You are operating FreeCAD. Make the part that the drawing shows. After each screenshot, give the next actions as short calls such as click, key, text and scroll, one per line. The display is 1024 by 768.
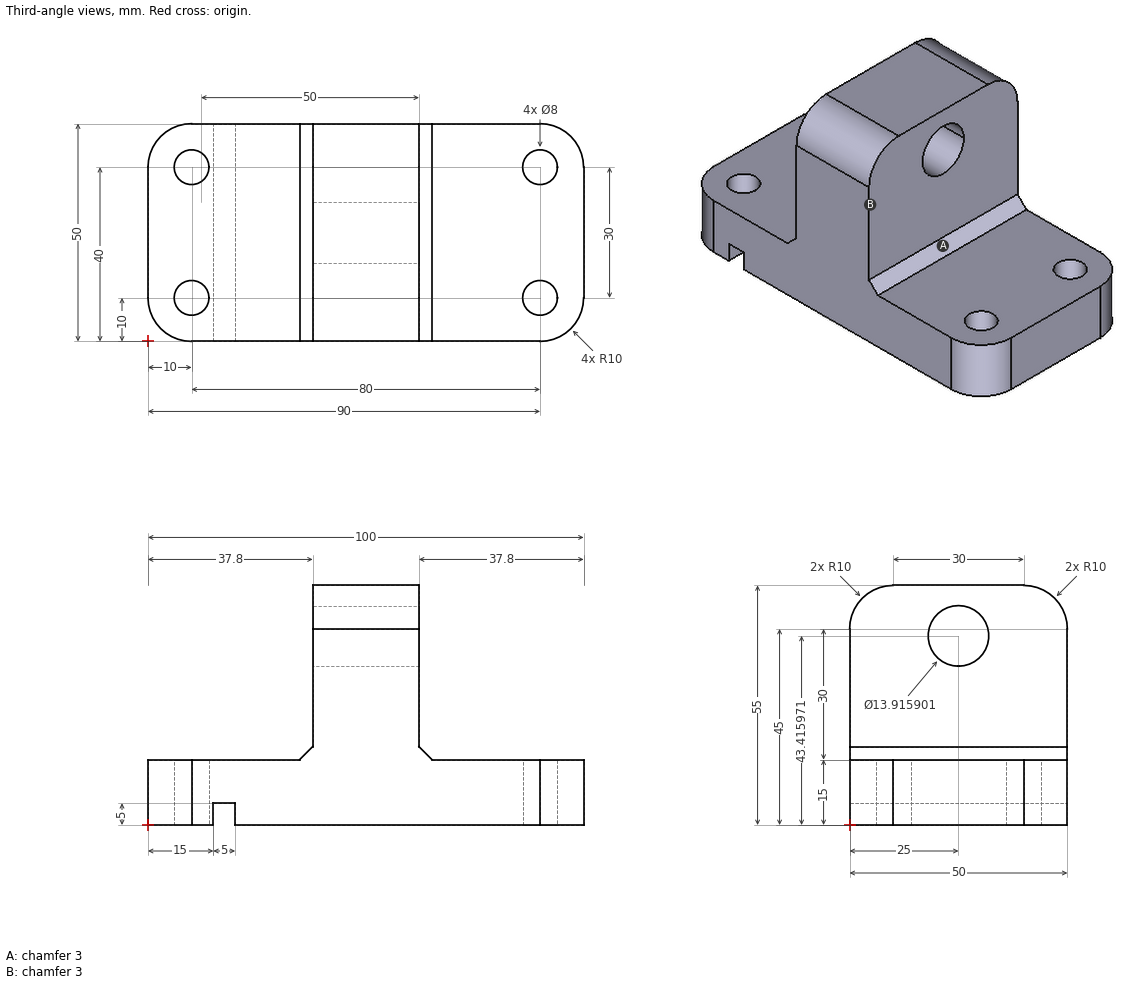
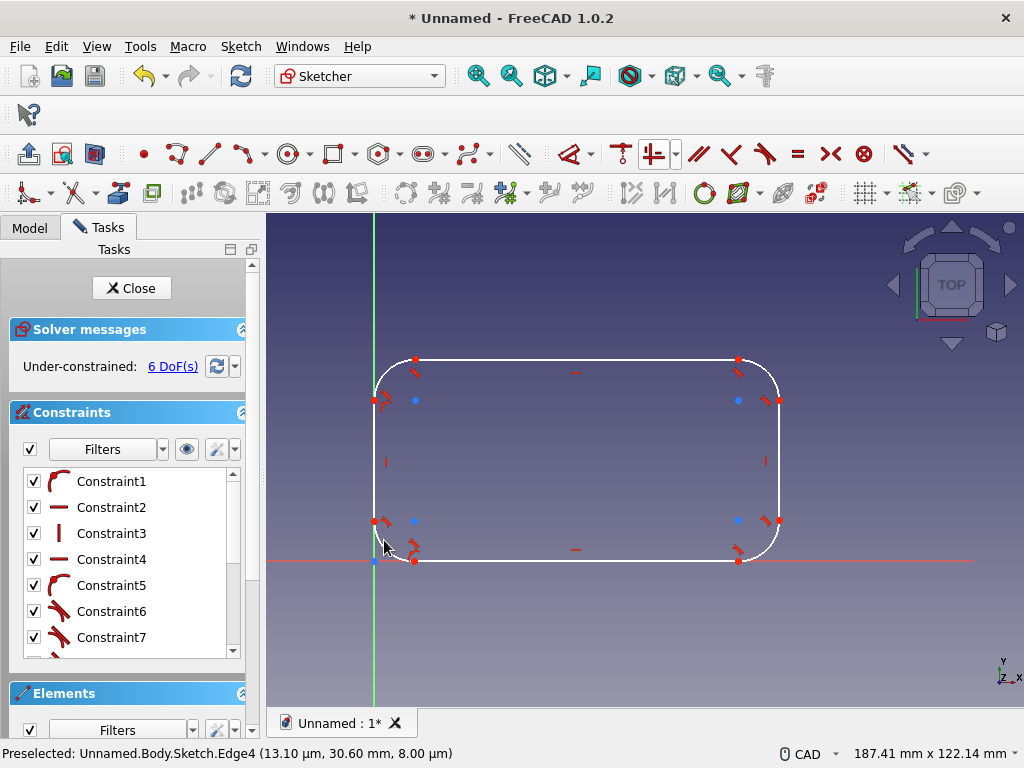
click(775, 539)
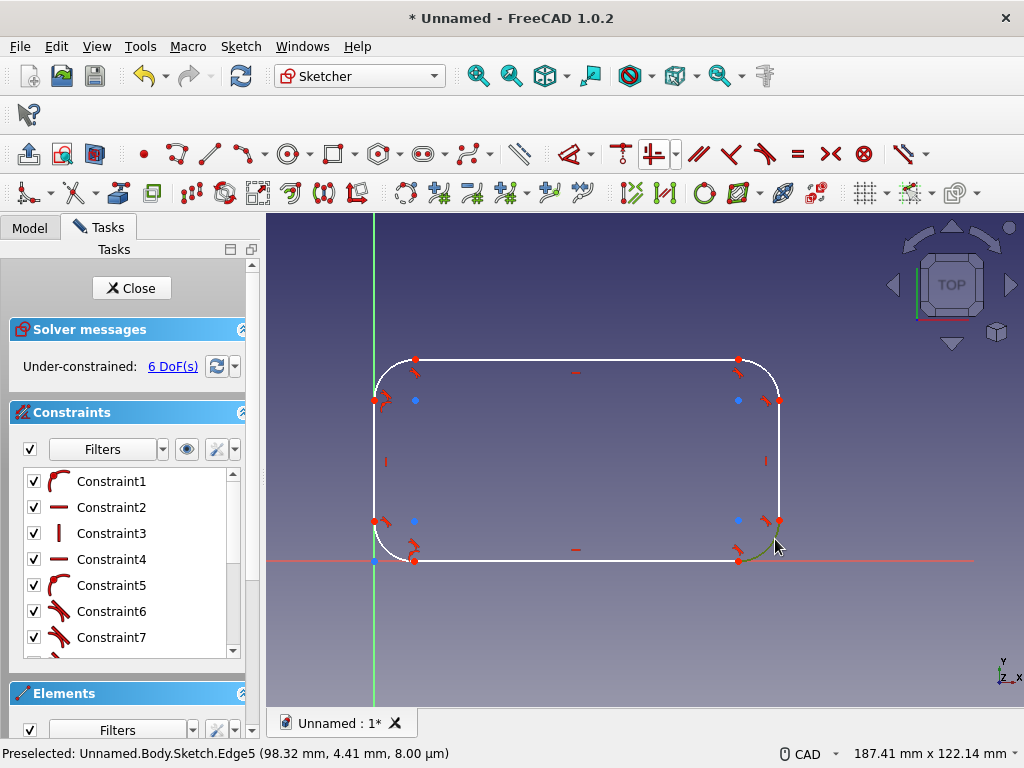
click(775, 382)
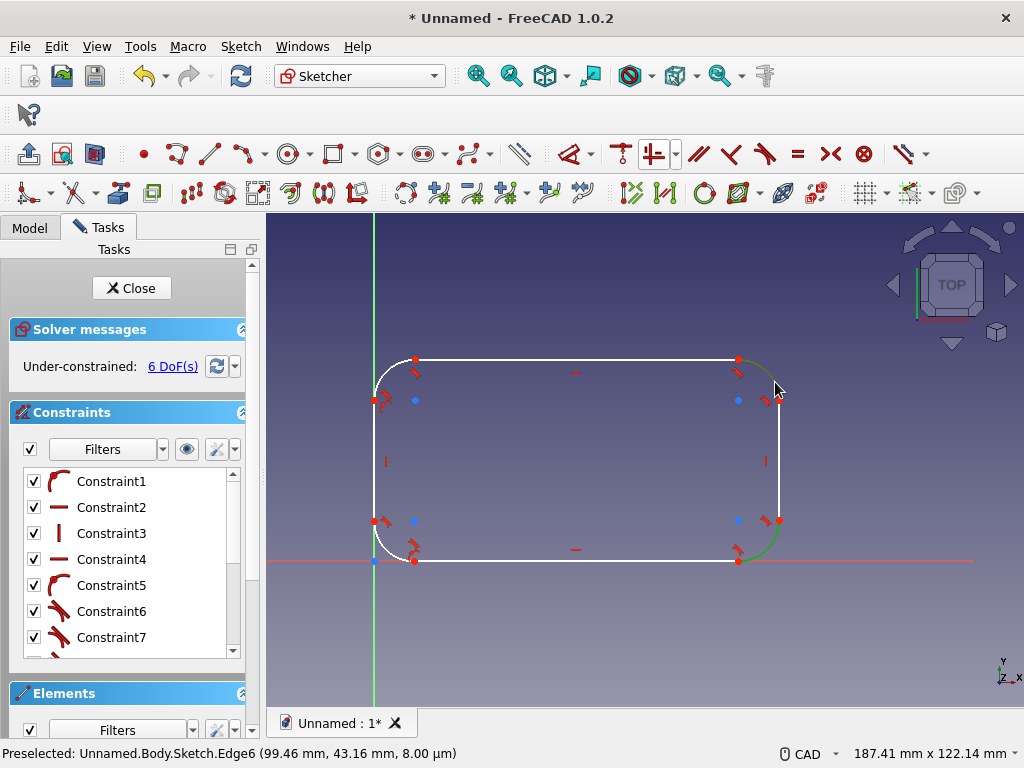
click(397, 364)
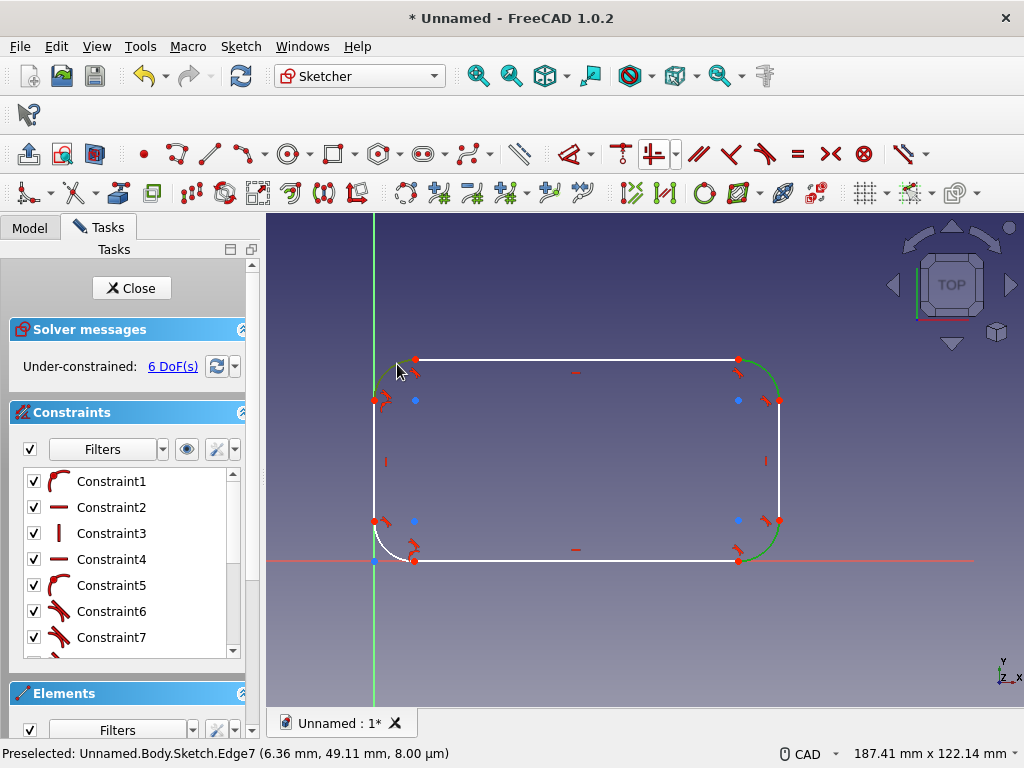
click(386, 550)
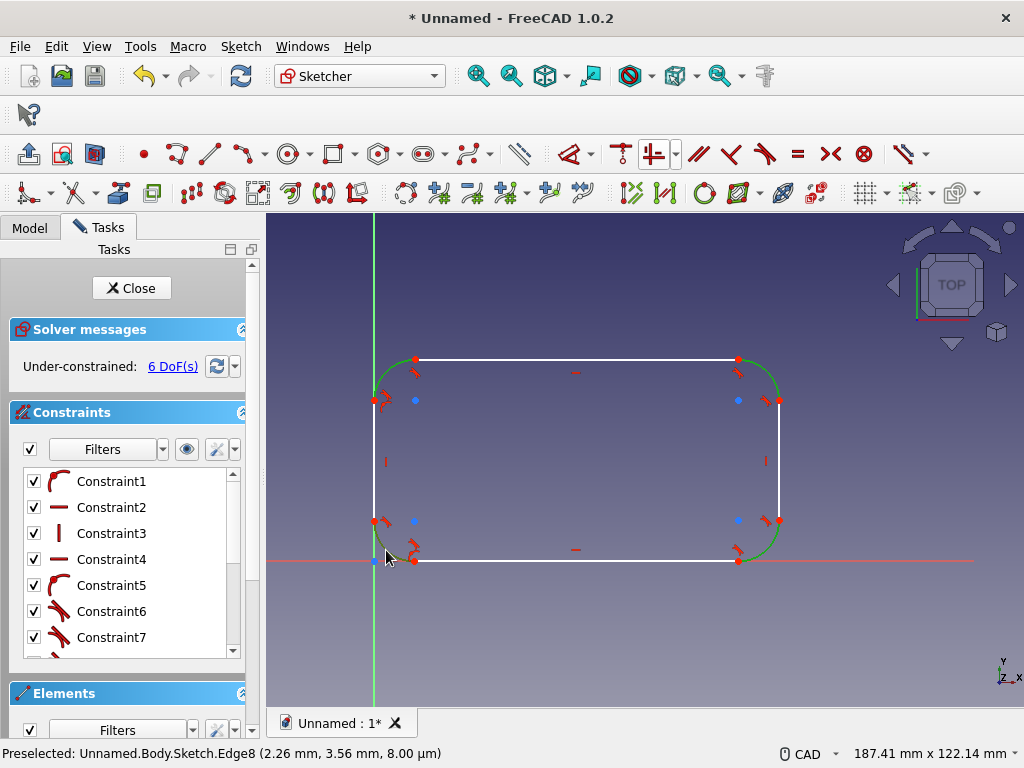
click(798, 154)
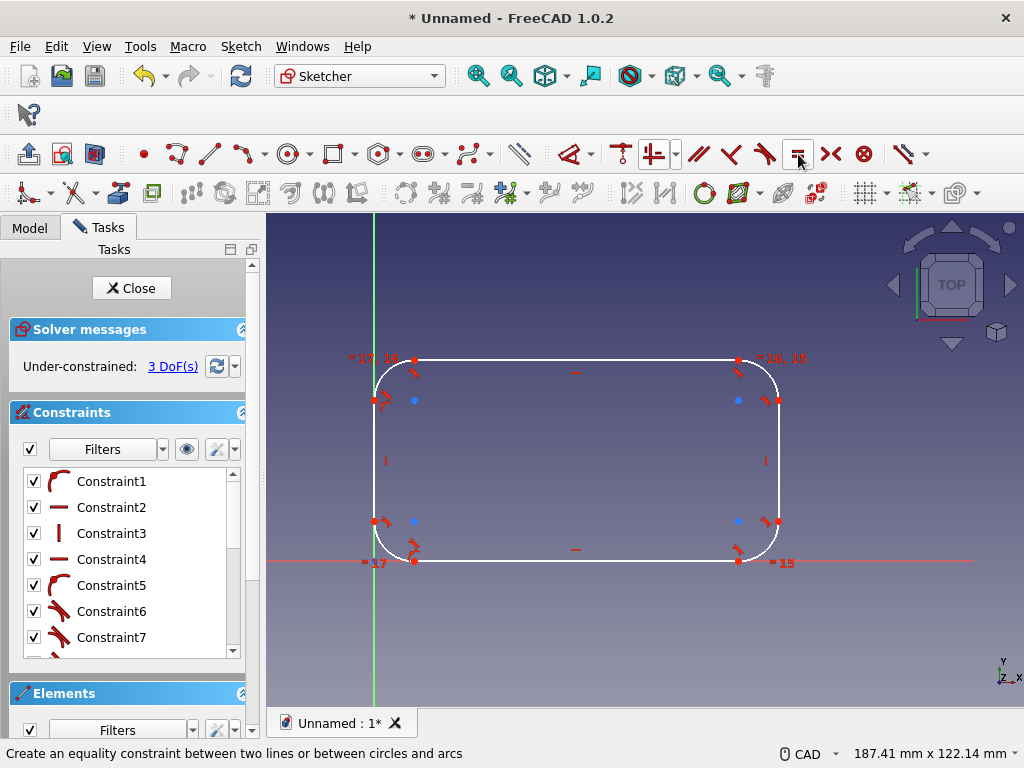
click(568, 154)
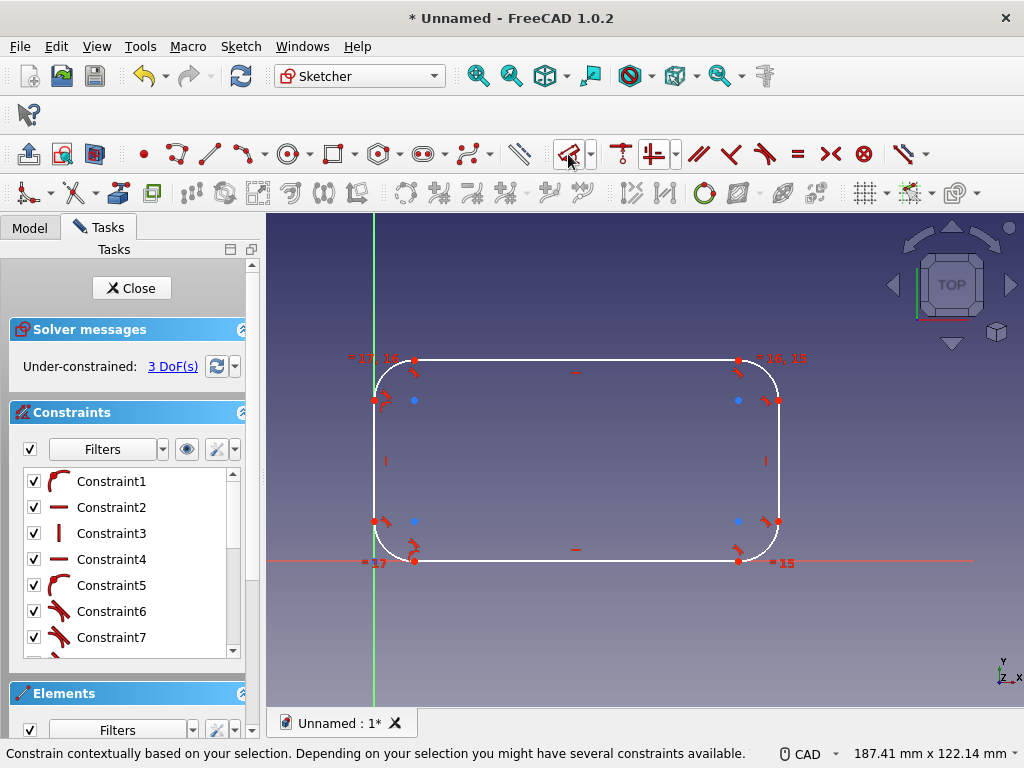
click(774, 539)
click(779, 580)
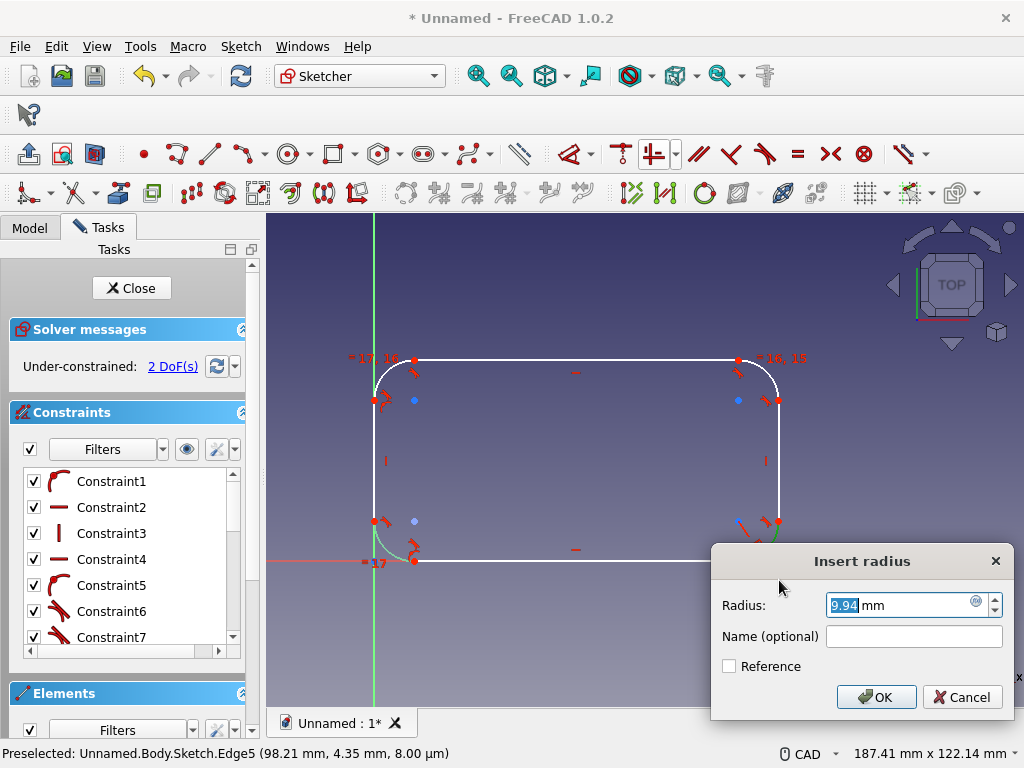
text(10)
key(Return)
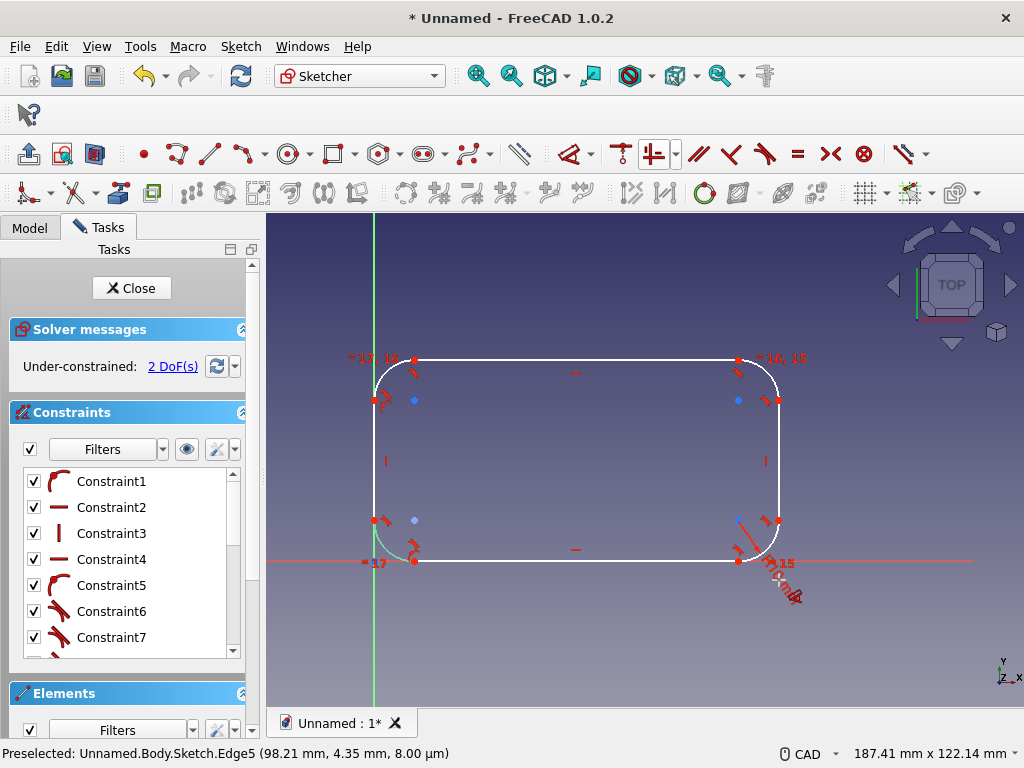
click(512, 561)
click(577, 595)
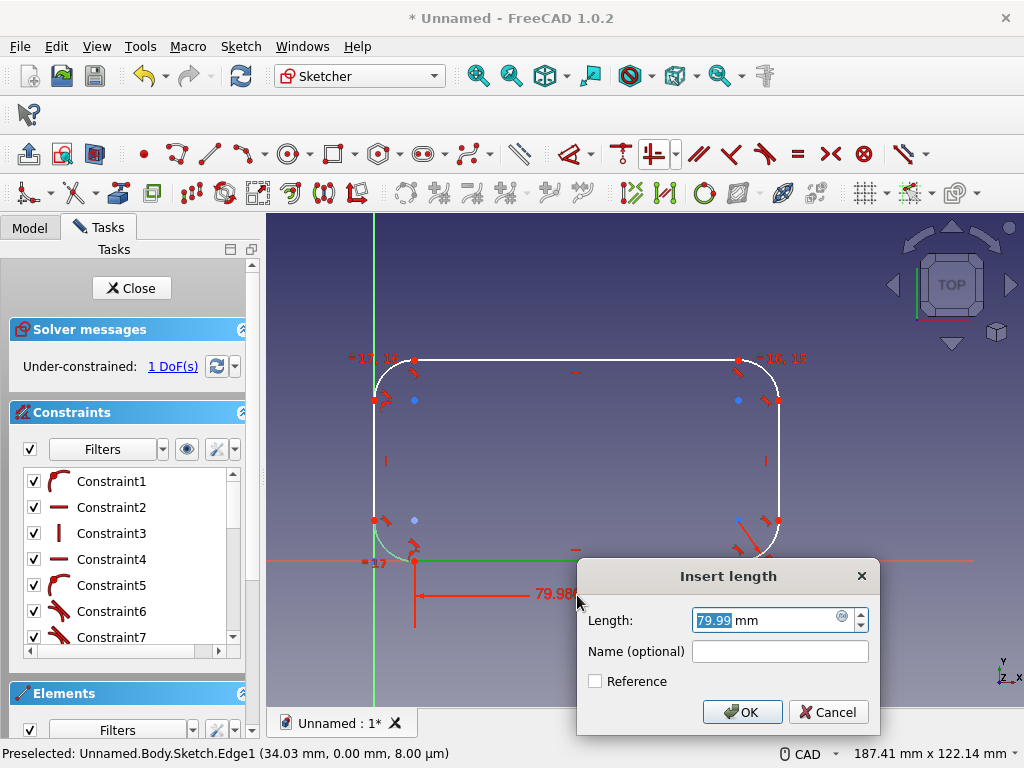
text(80)
key(Return)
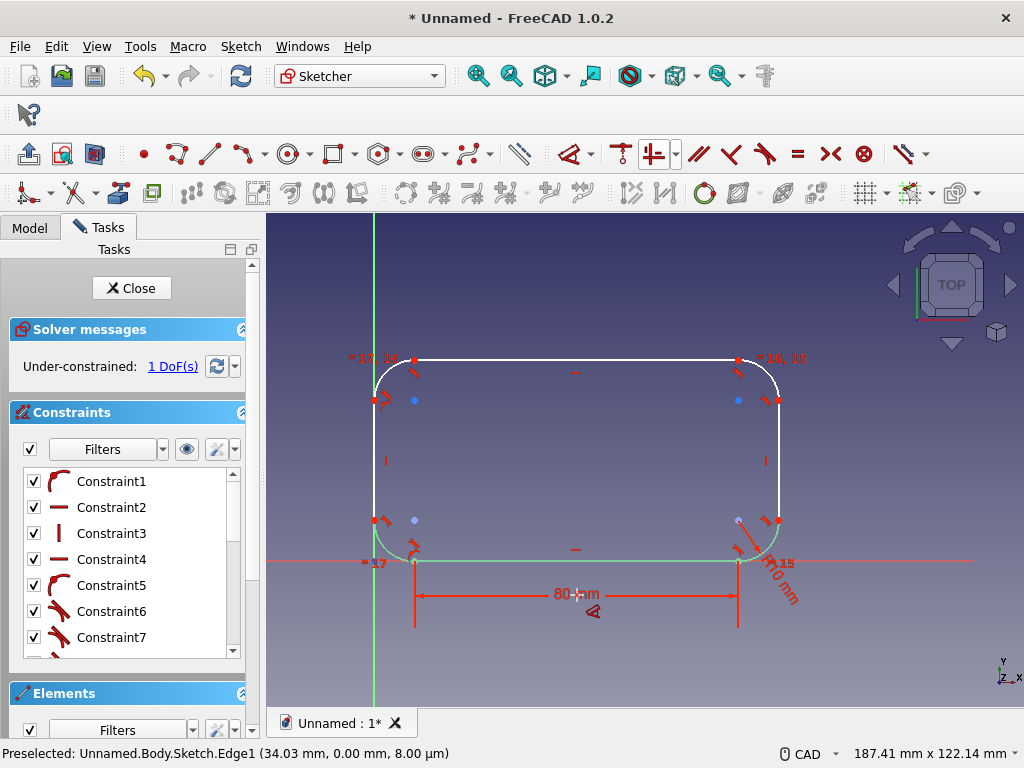
click(779, 485)
click(813, 461)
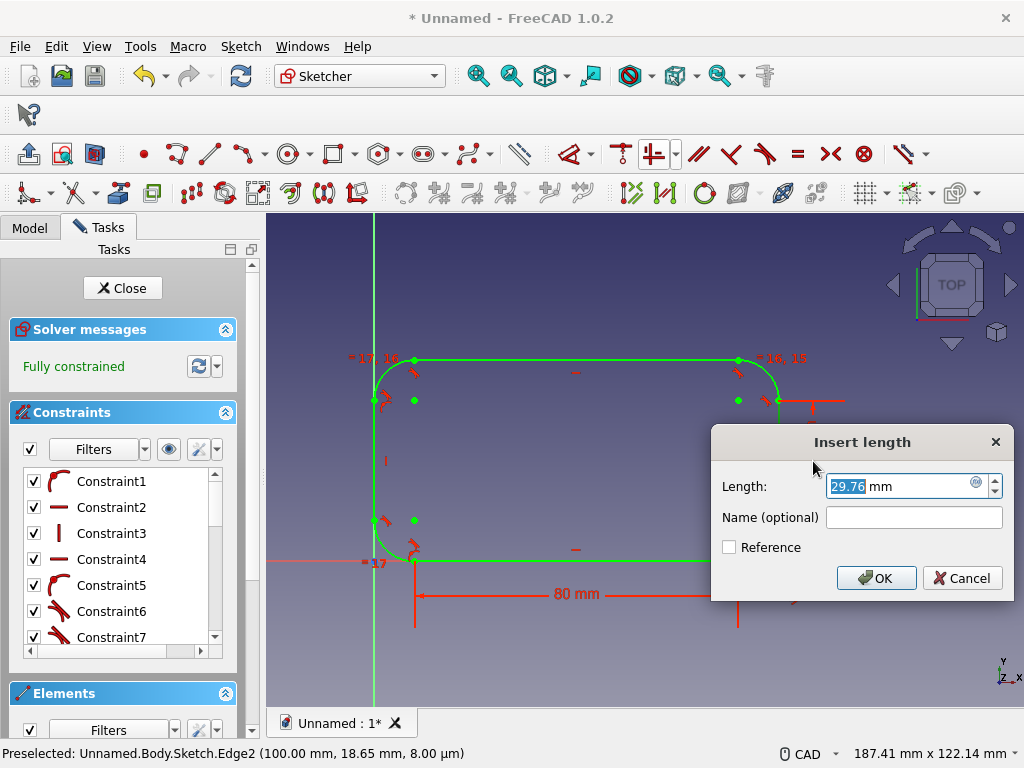
text(30)
key(Return)
key(Escape)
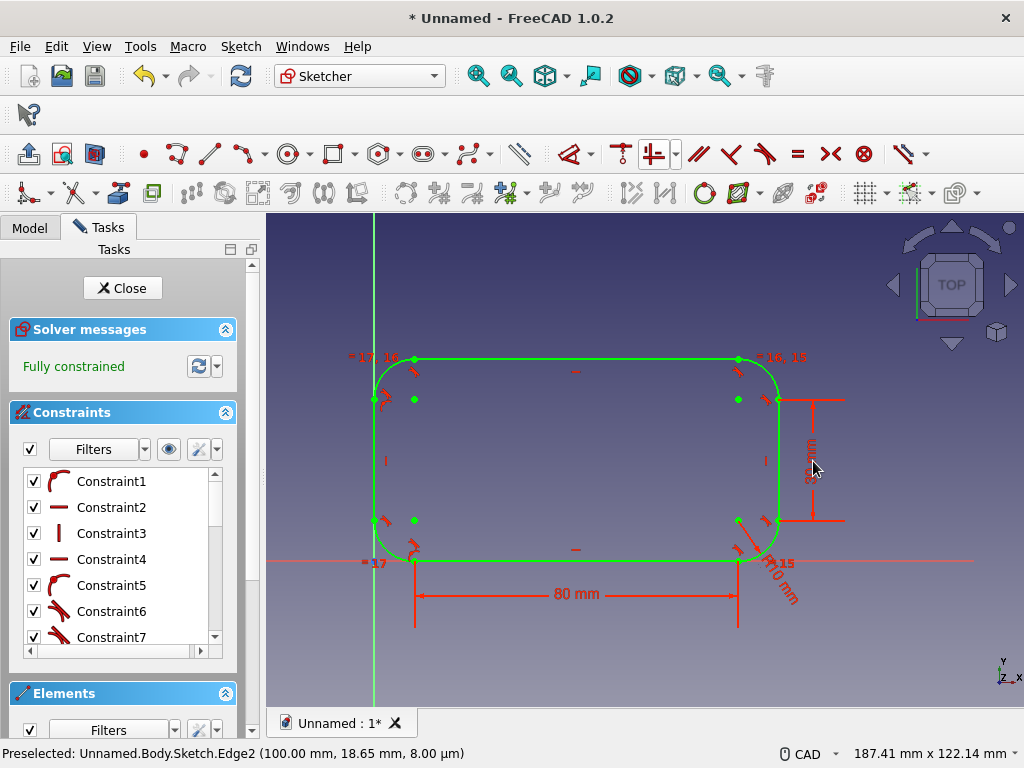
click(123, 288)